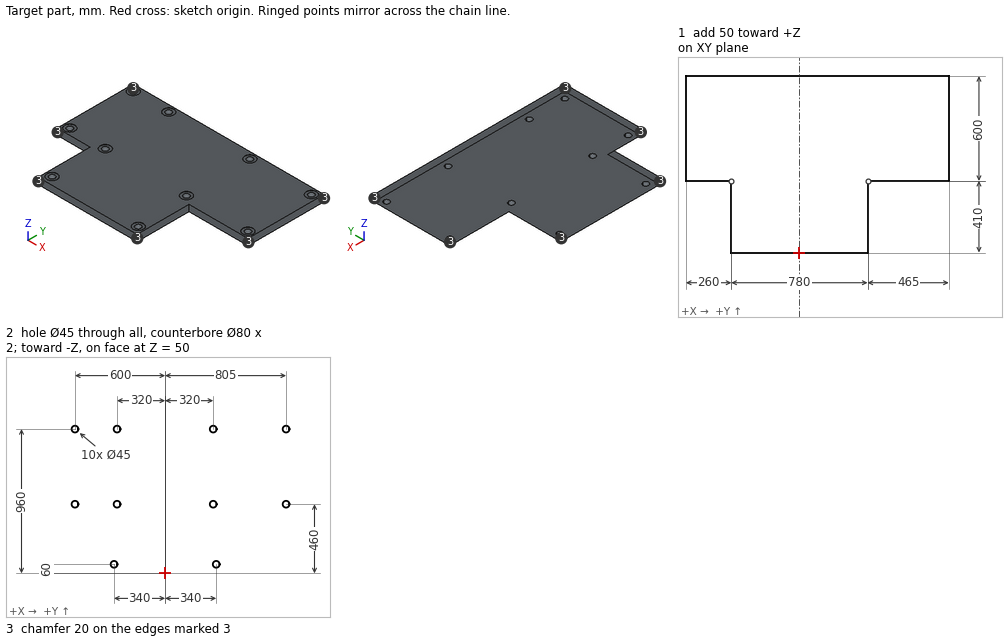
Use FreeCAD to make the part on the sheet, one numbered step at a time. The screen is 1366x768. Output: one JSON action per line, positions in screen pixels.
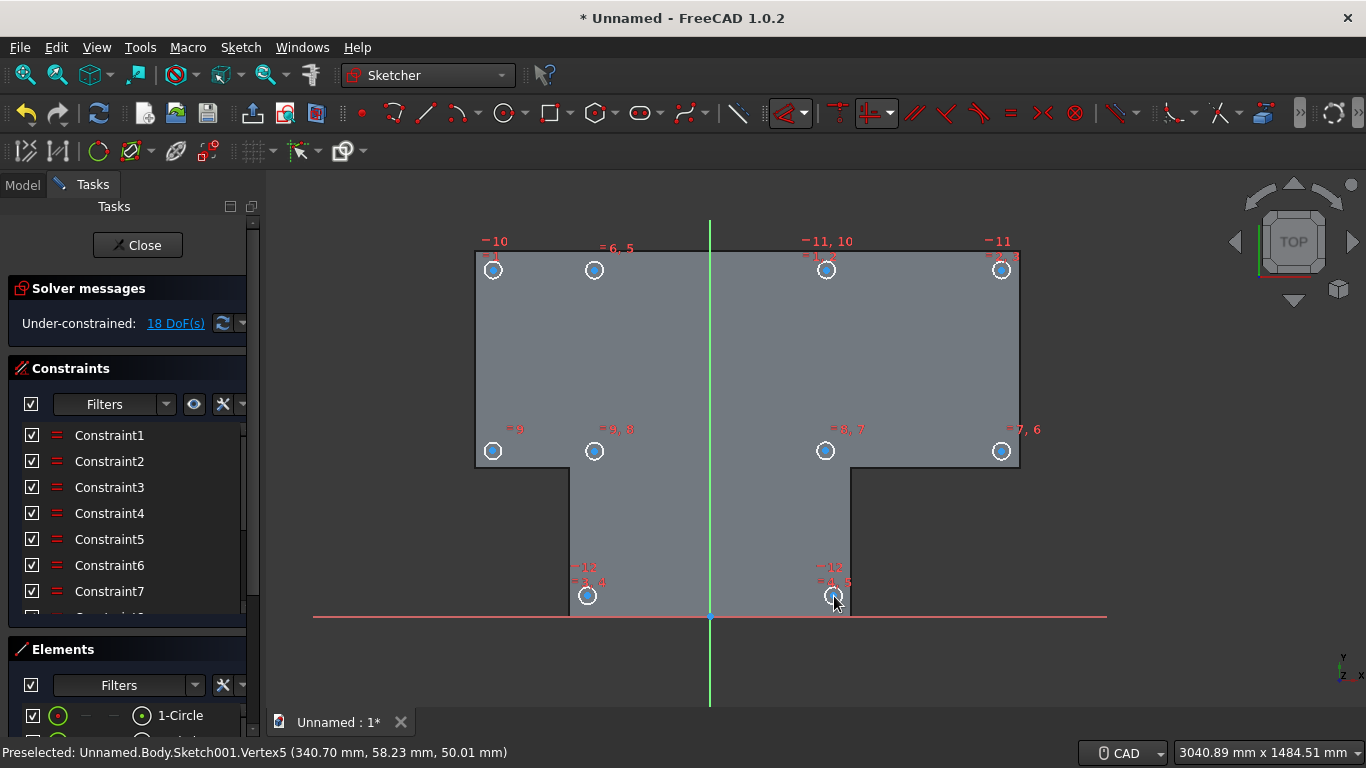
{"action": "left_click", "coordinate": [493, 270]}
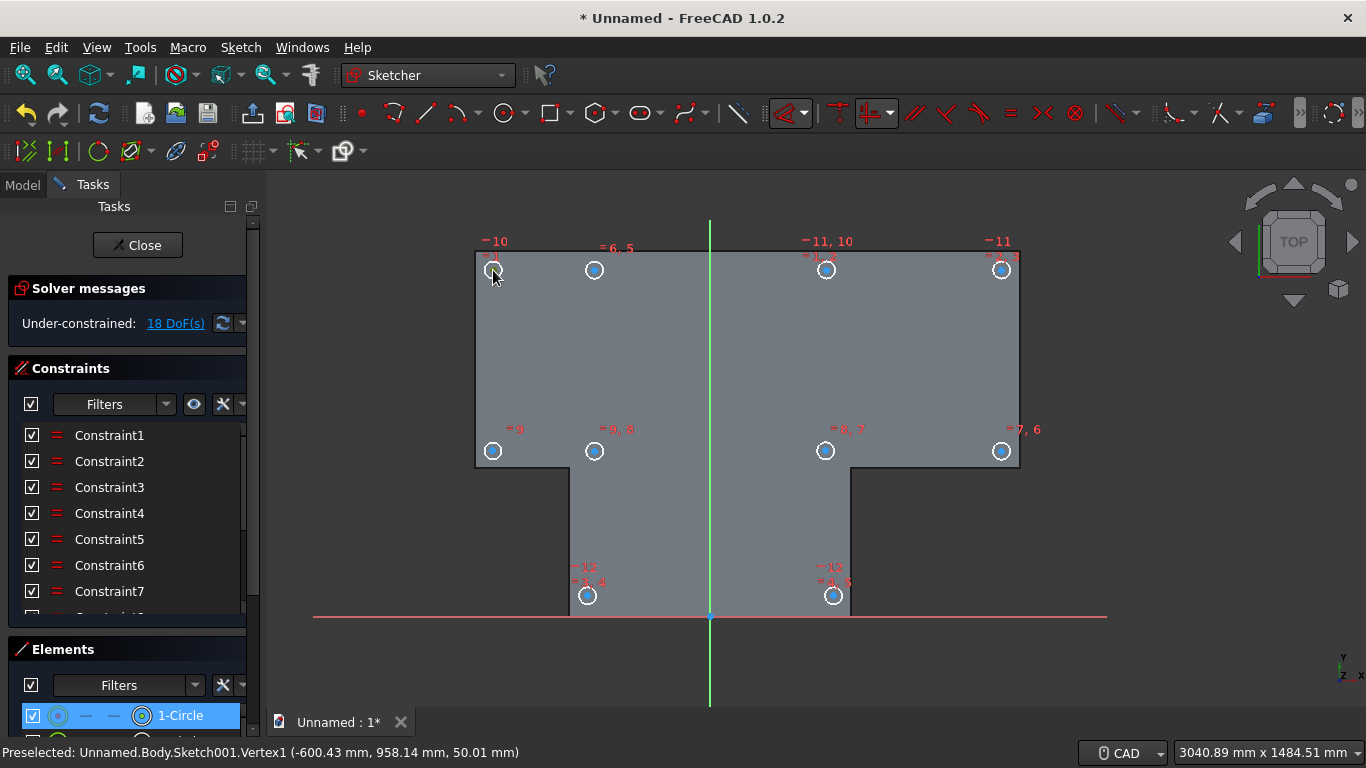
{"action": "left_click", "coordinate": [595, 270]}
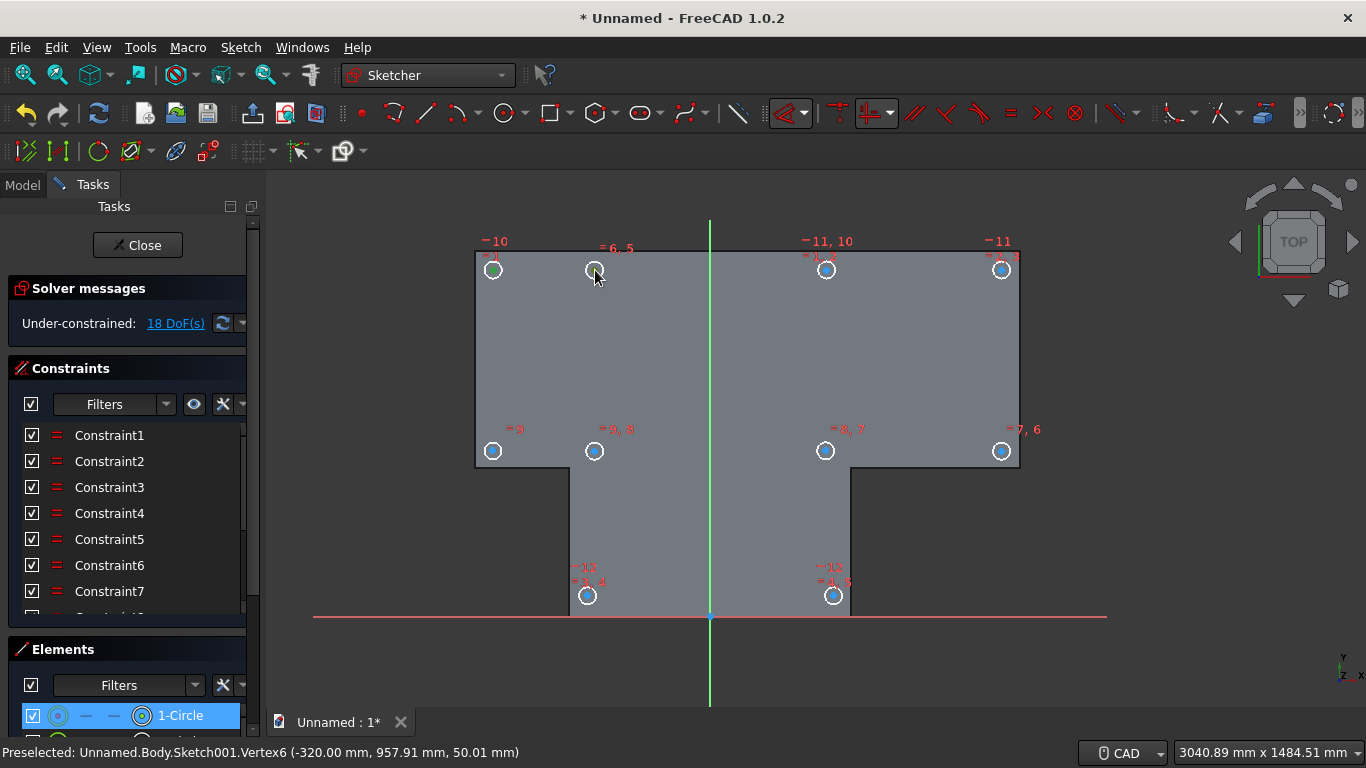
{"action": "key", "text": "h"}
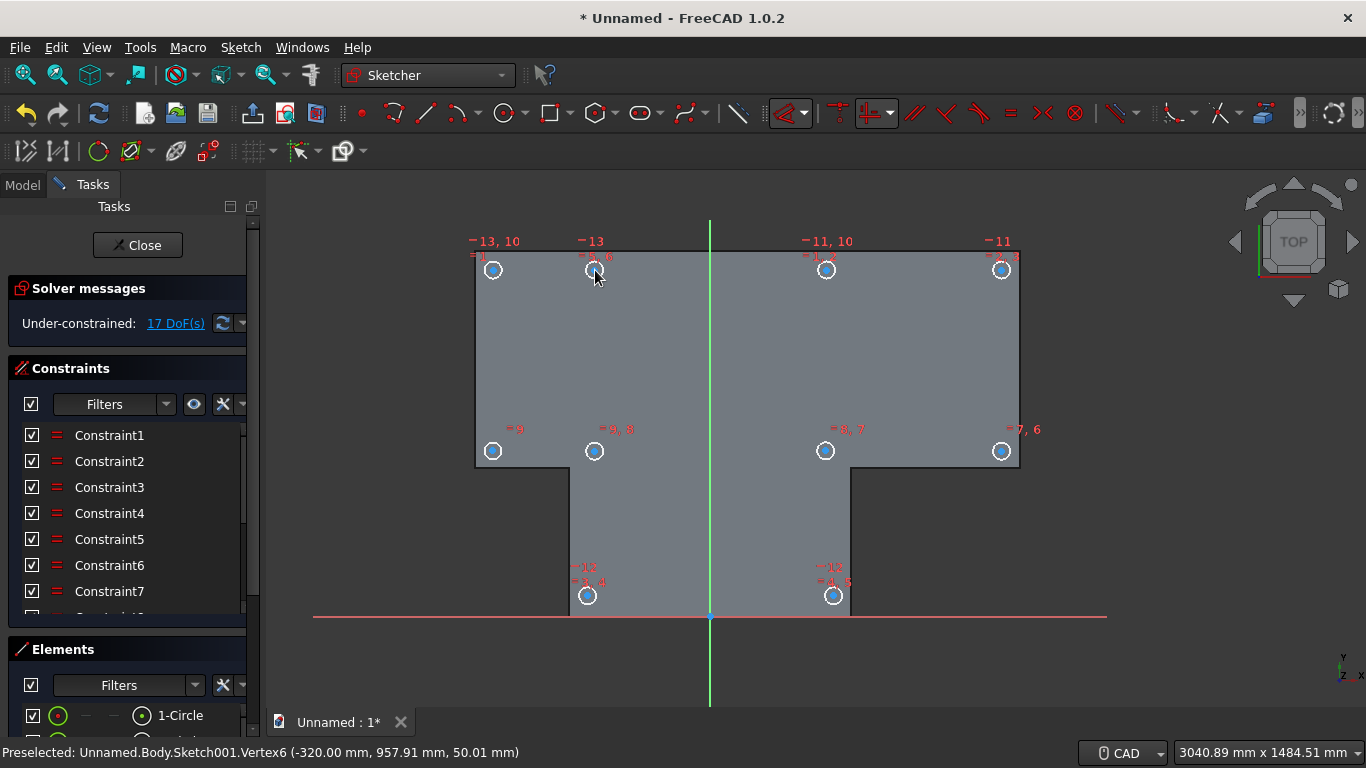
{"action": "left_click", "coordinate": [1002, 270]}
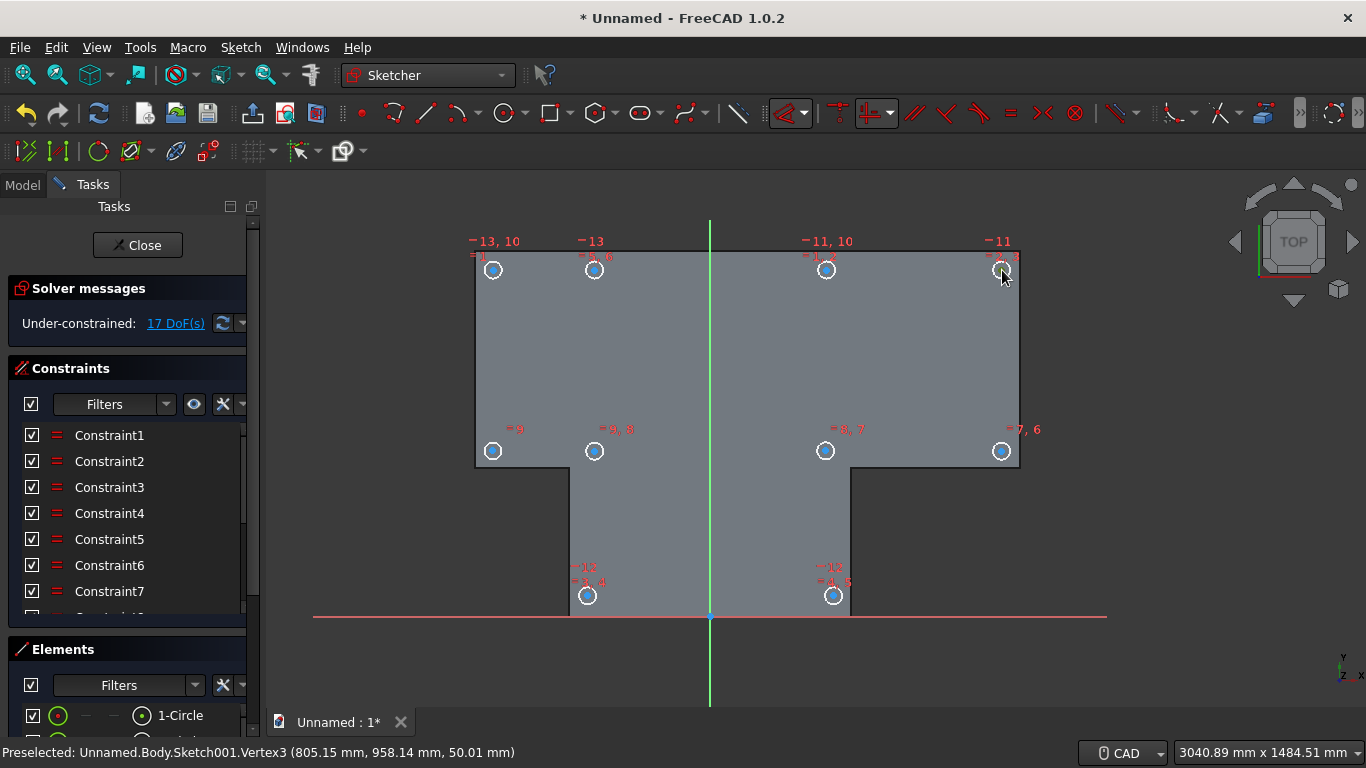
{"action": "left_click", "coordinate": [1002, 451]}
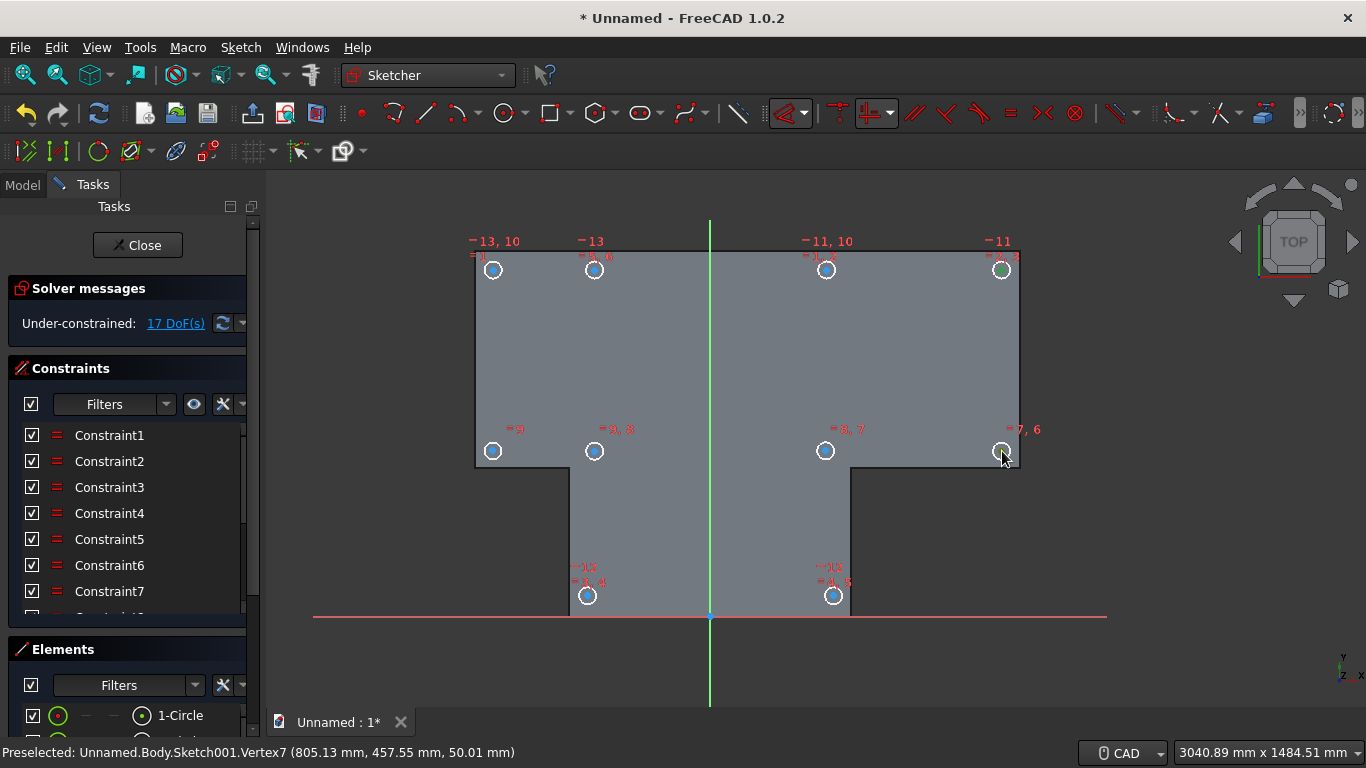
{"action": "left_click", "coordinate": [892, 114]}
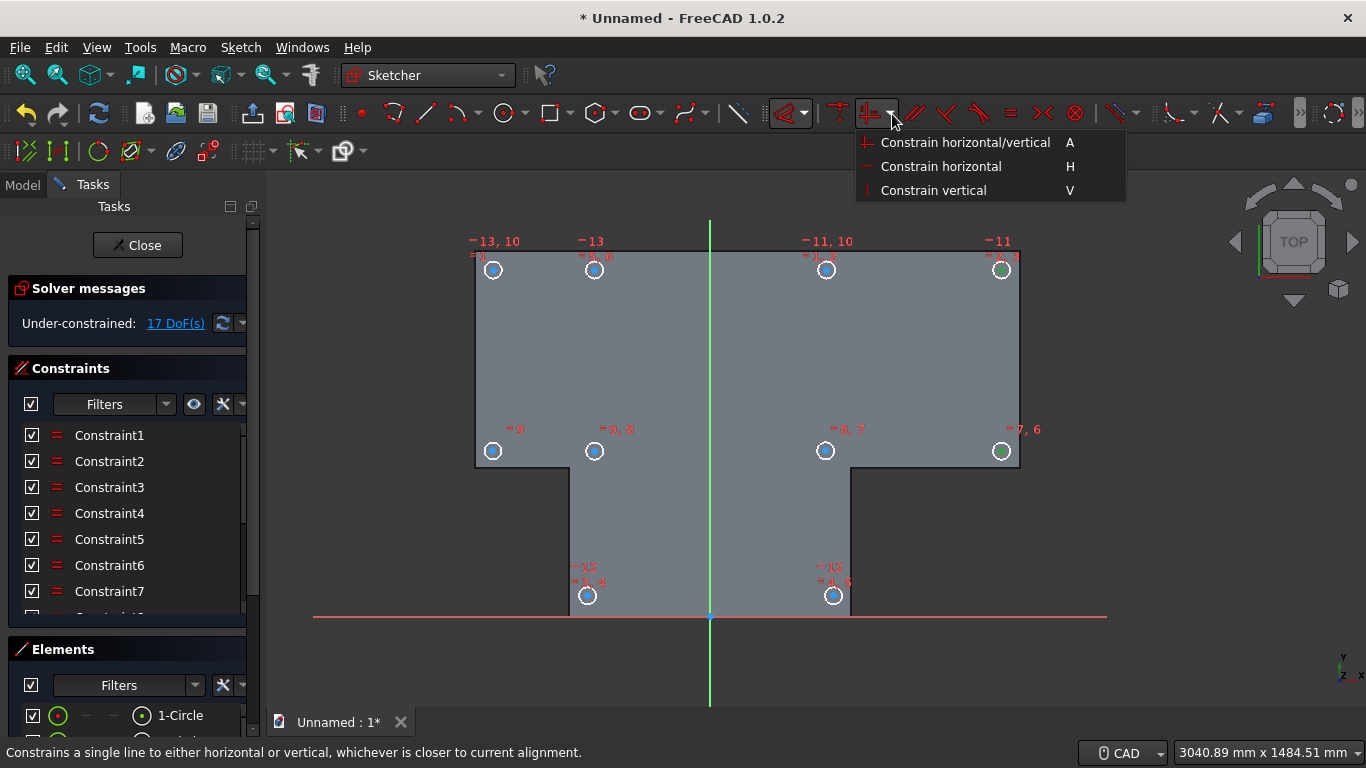
{"action": "left_click", "coordinate": [991, 190]}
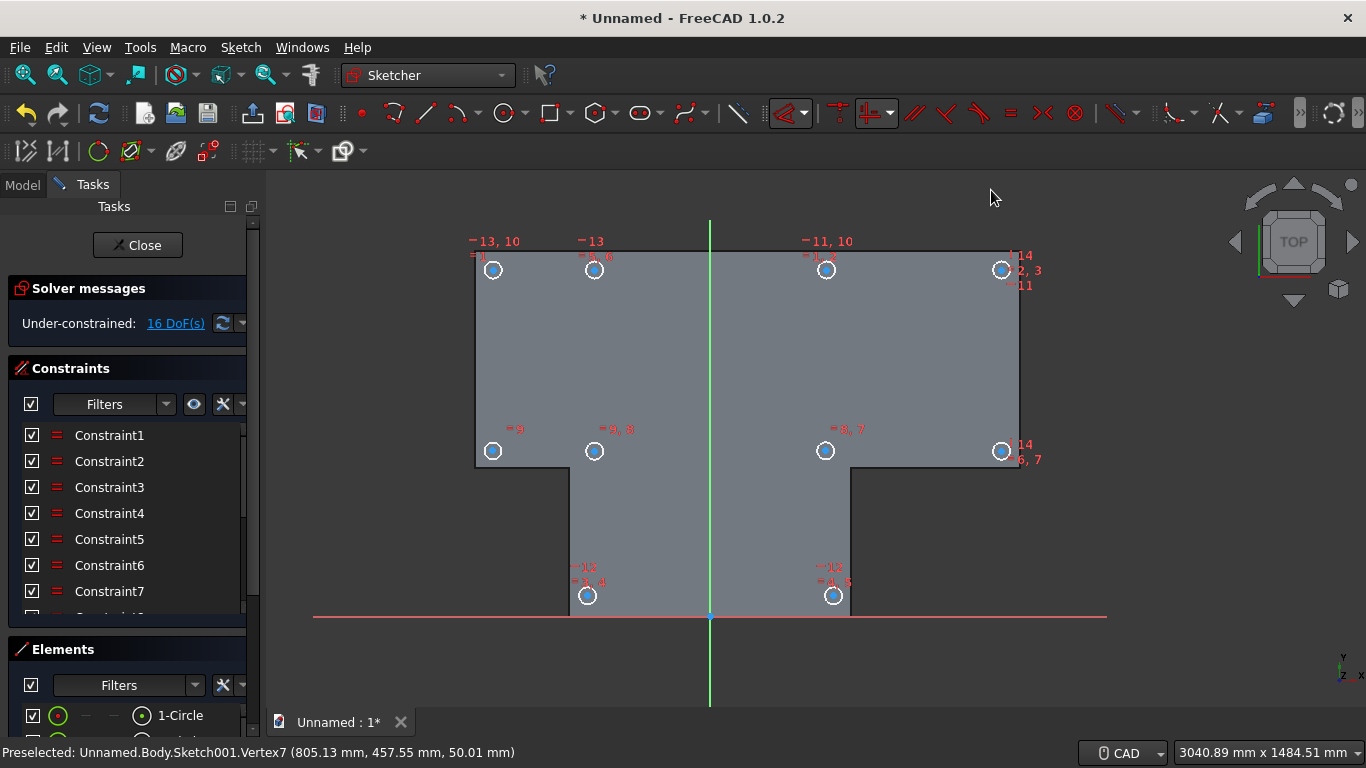
{"action": "left_click", "coordinate": [827, 270]}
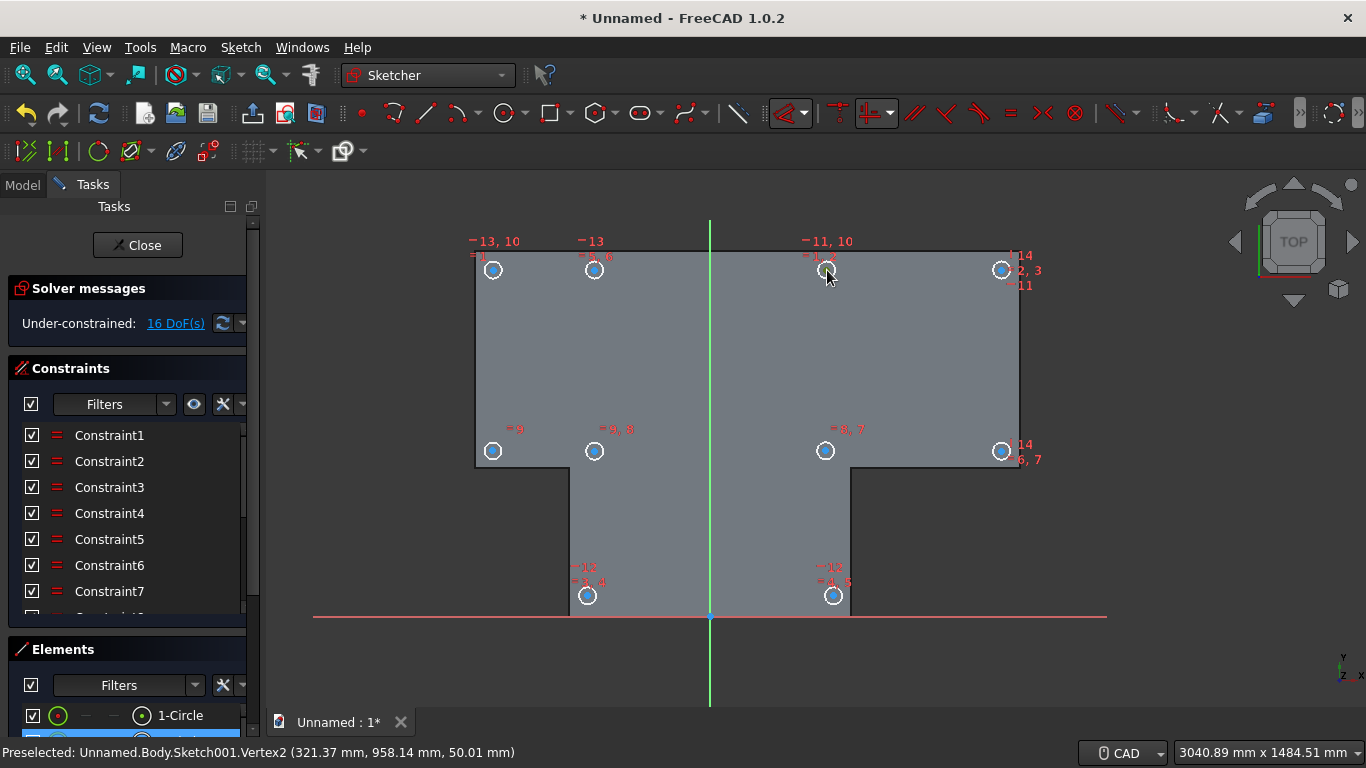
{"action": "left_click", "coordinate": [826, 451]}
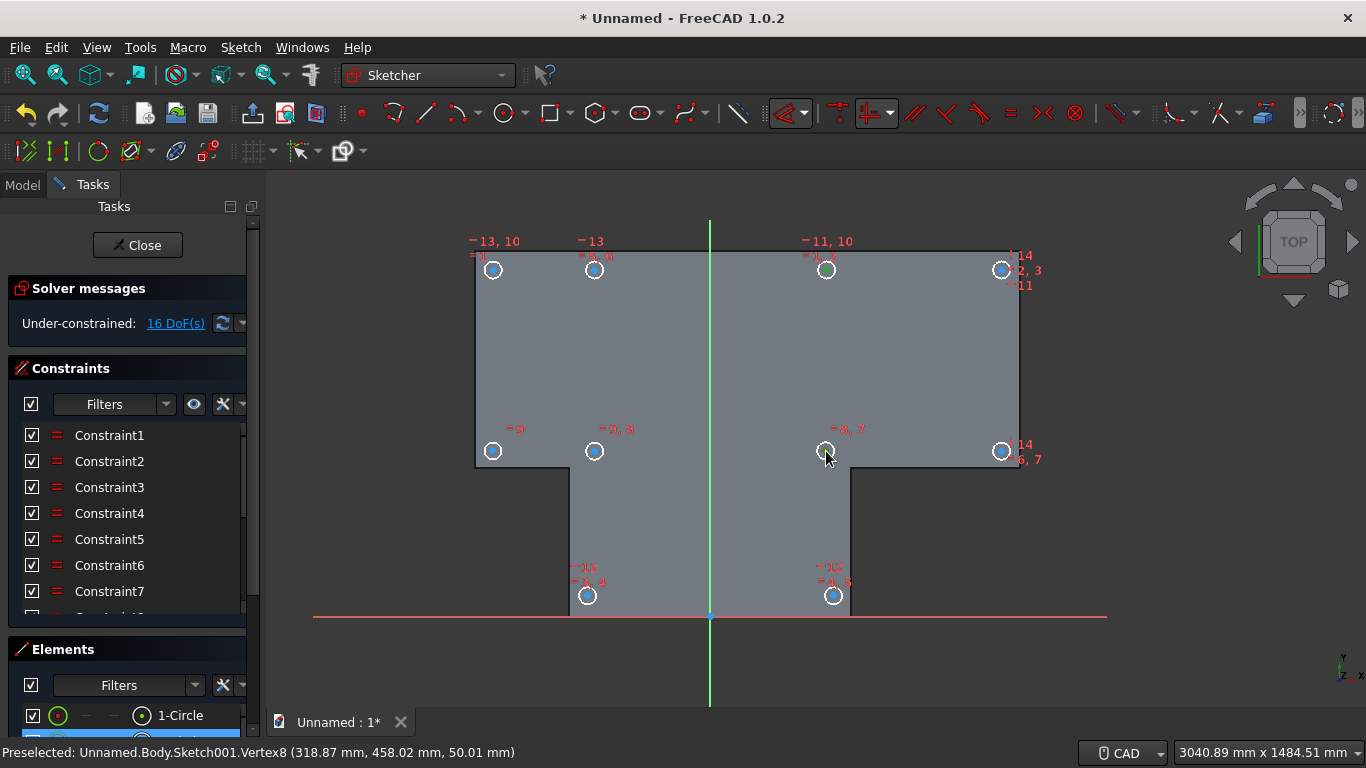
{"action": "key", "text": "v"}